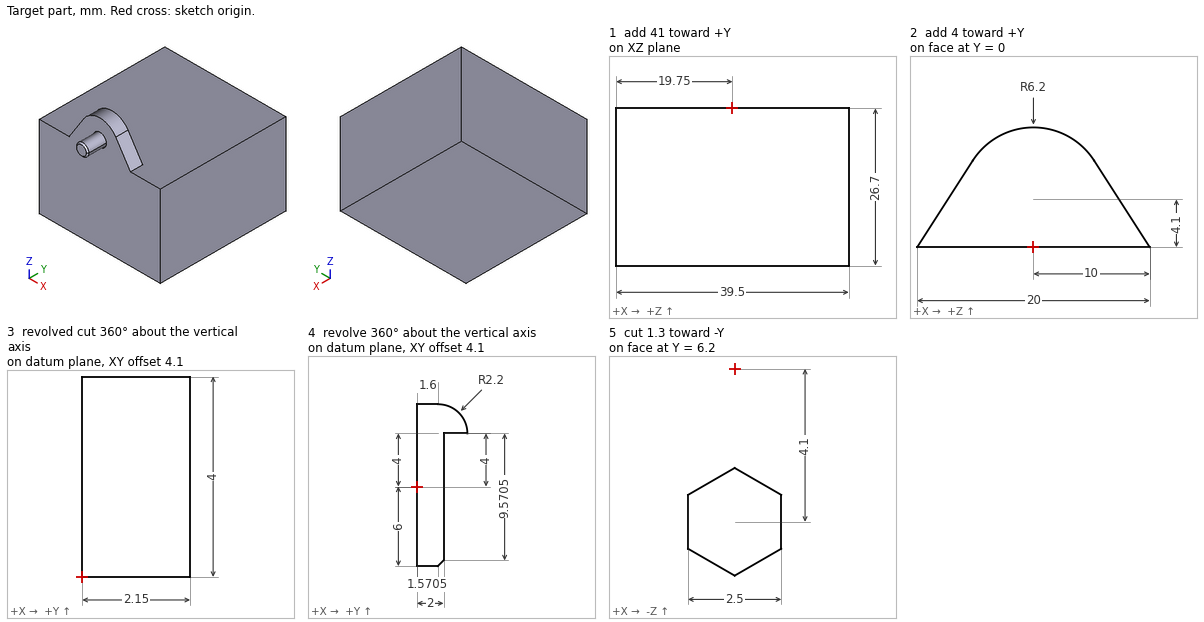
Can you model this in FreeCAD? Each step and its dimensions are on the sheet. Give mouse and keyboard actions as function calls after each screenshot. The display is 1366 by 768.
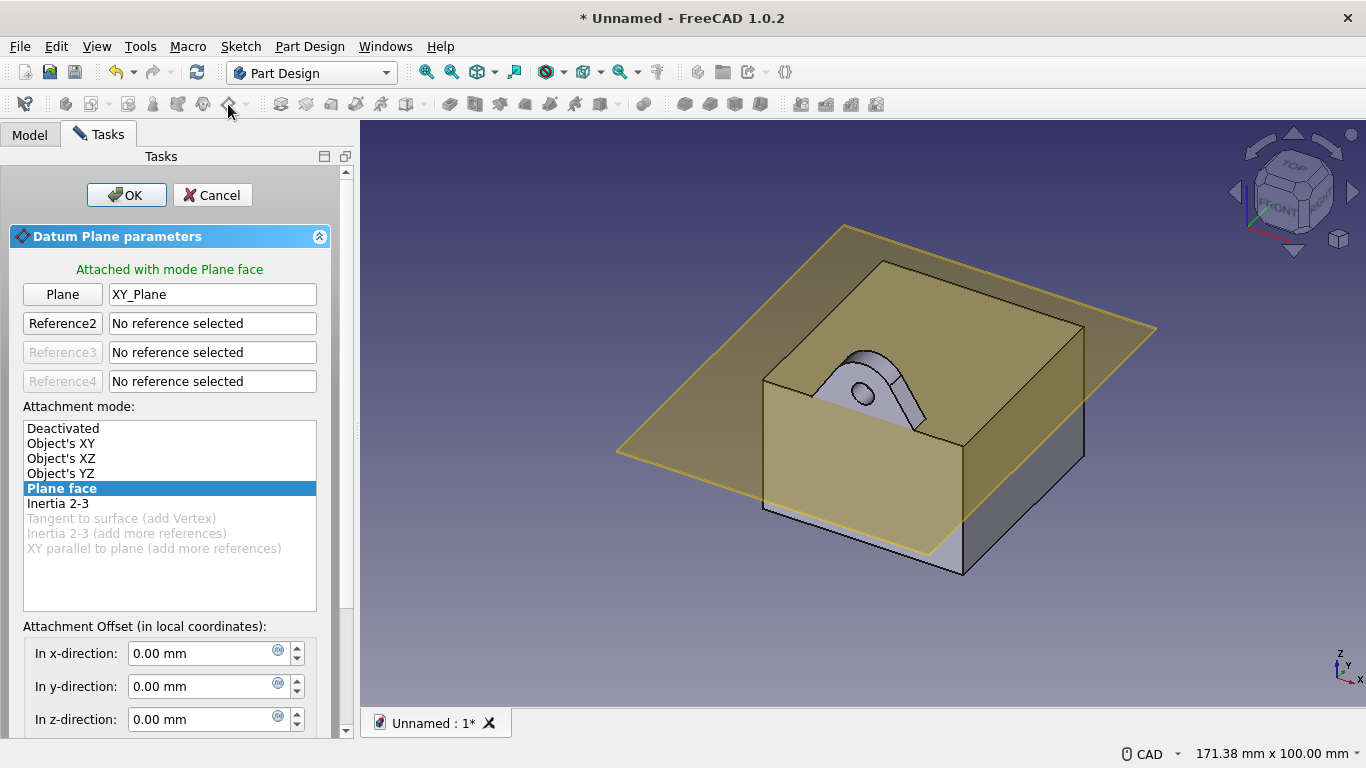
triple_click(210, 720)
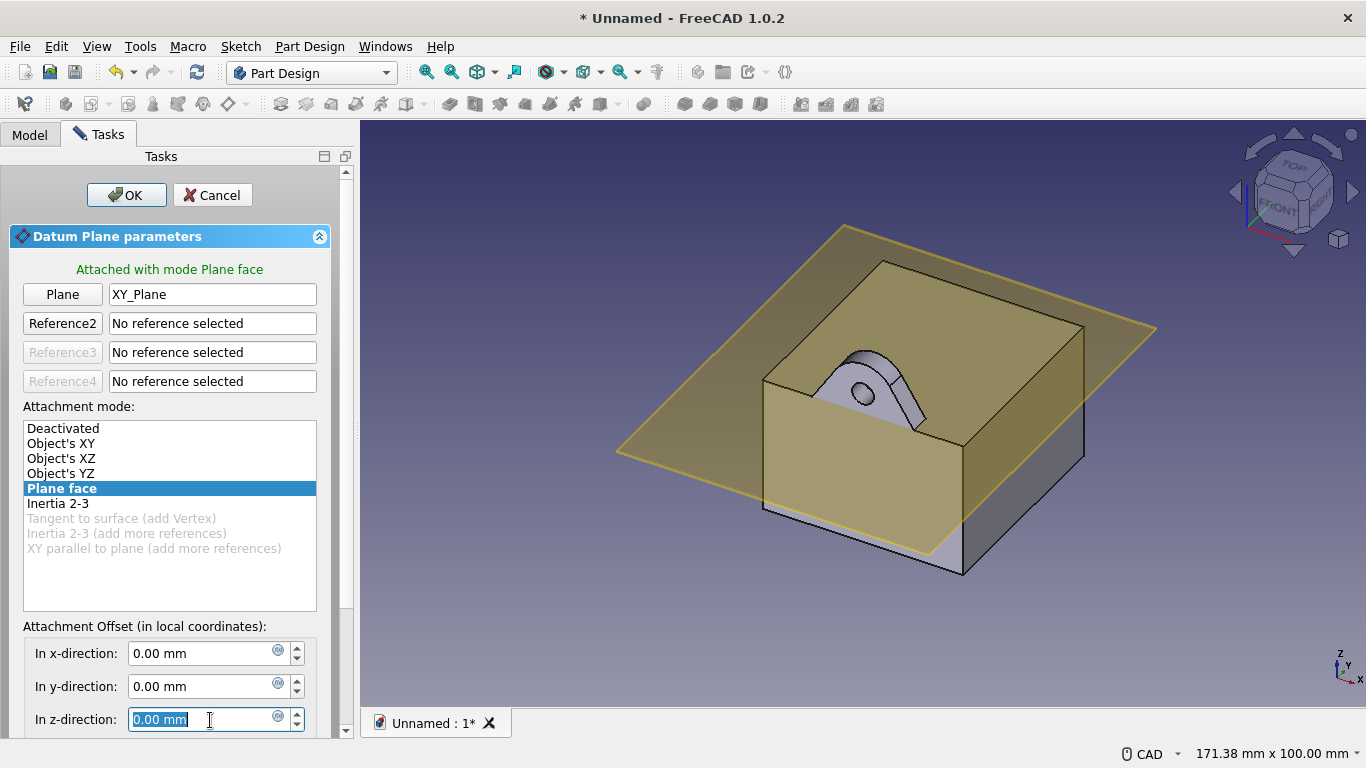
text(4.1)
key(Tab)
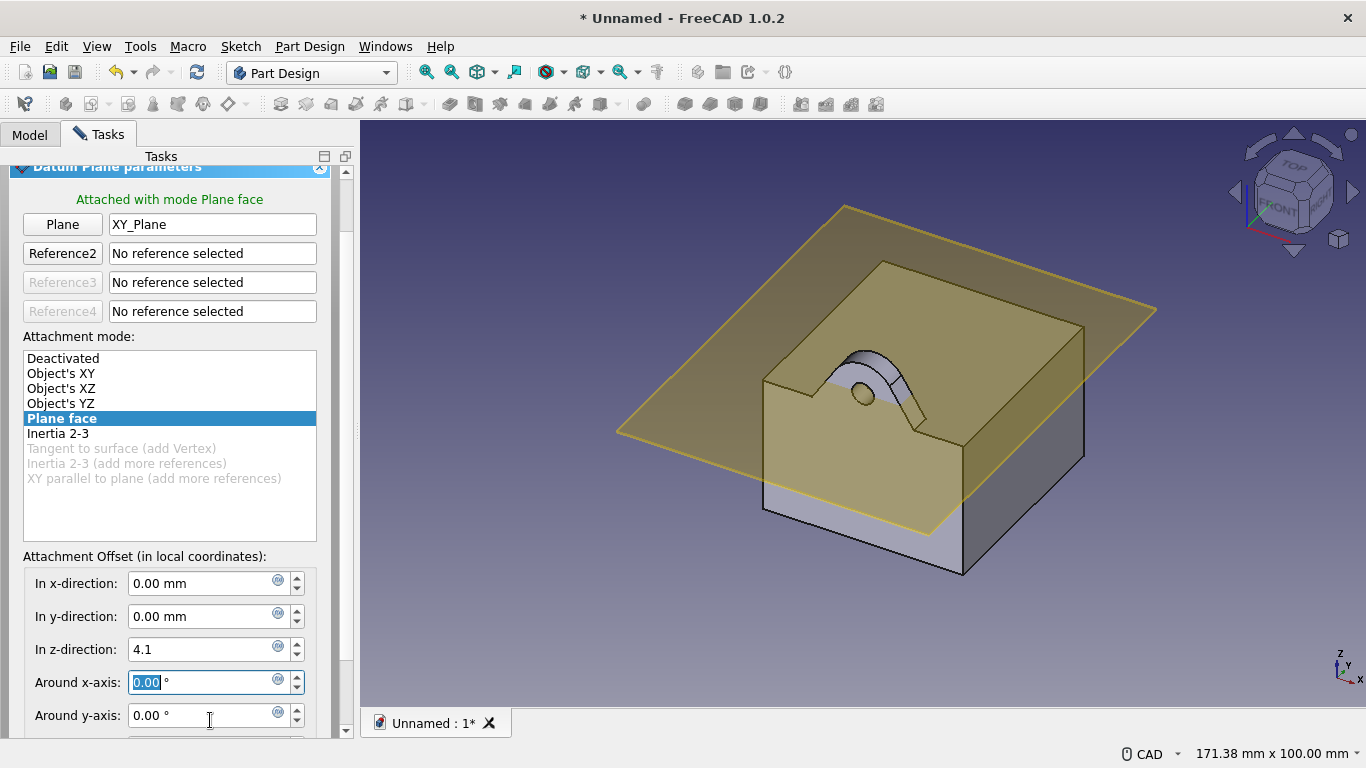
scroll(346, 452, up, 2)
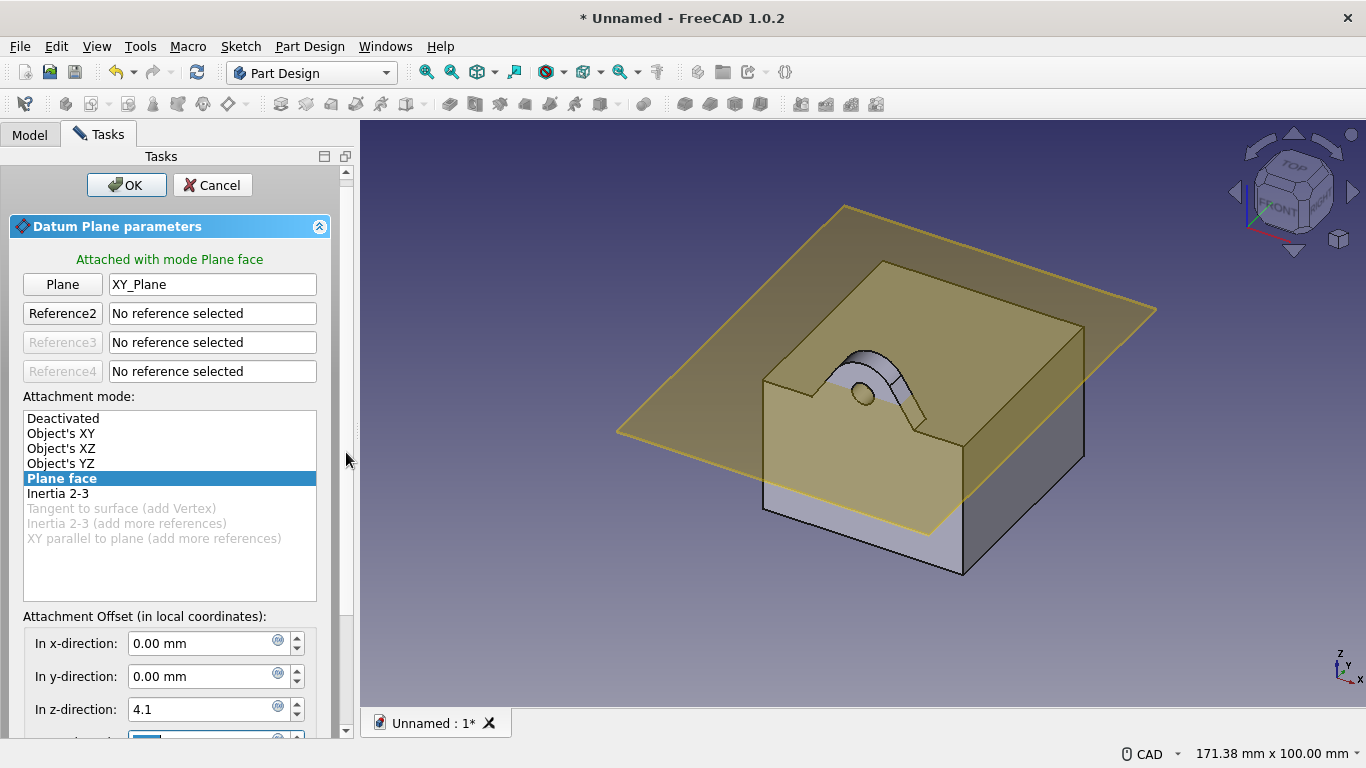
click(127, 195)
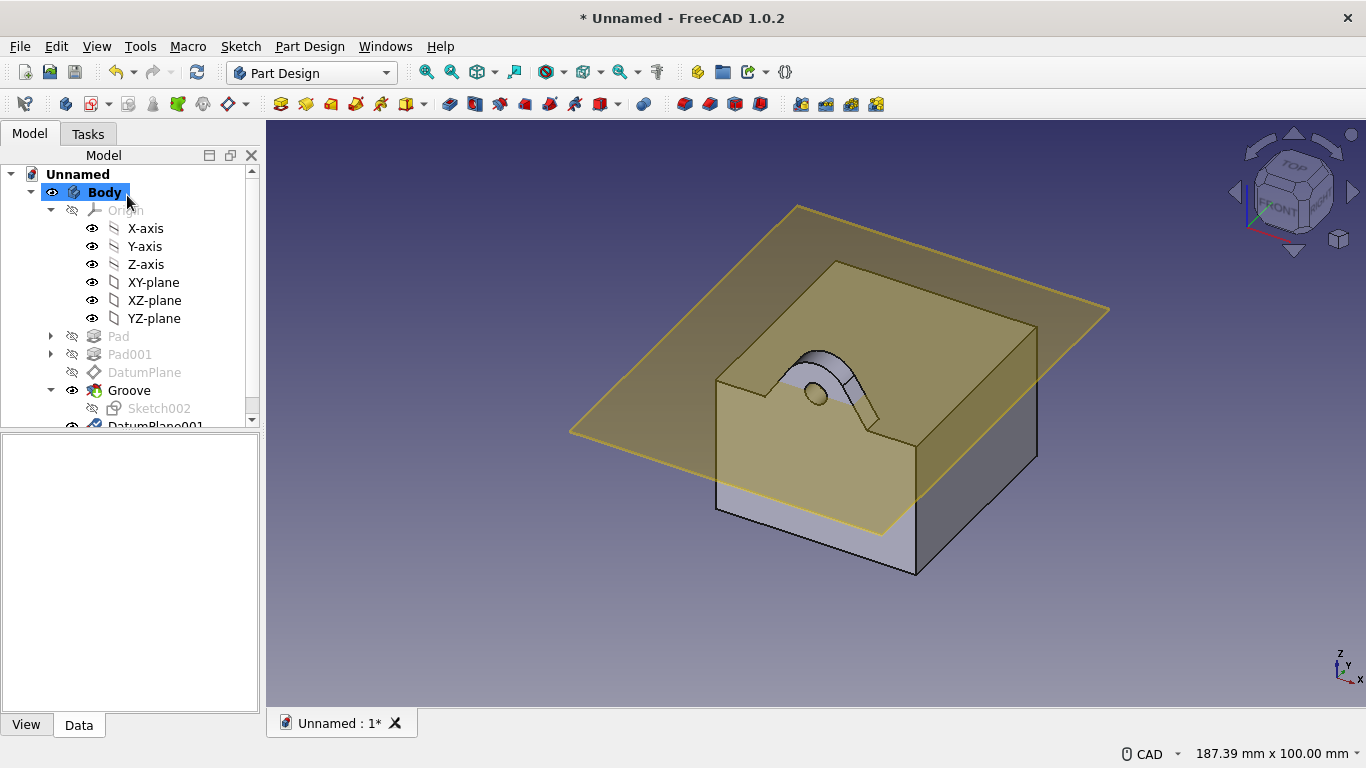
click(117, 426)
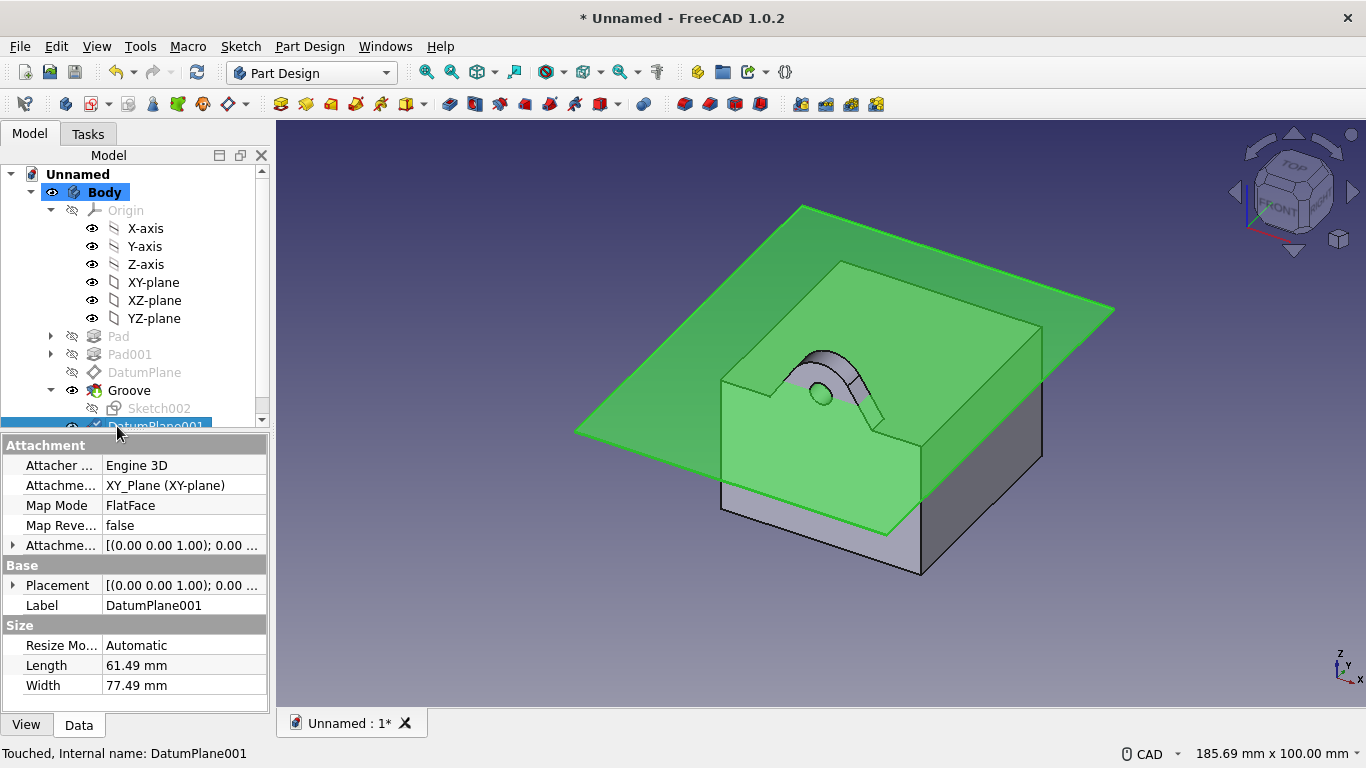
click(90, 104)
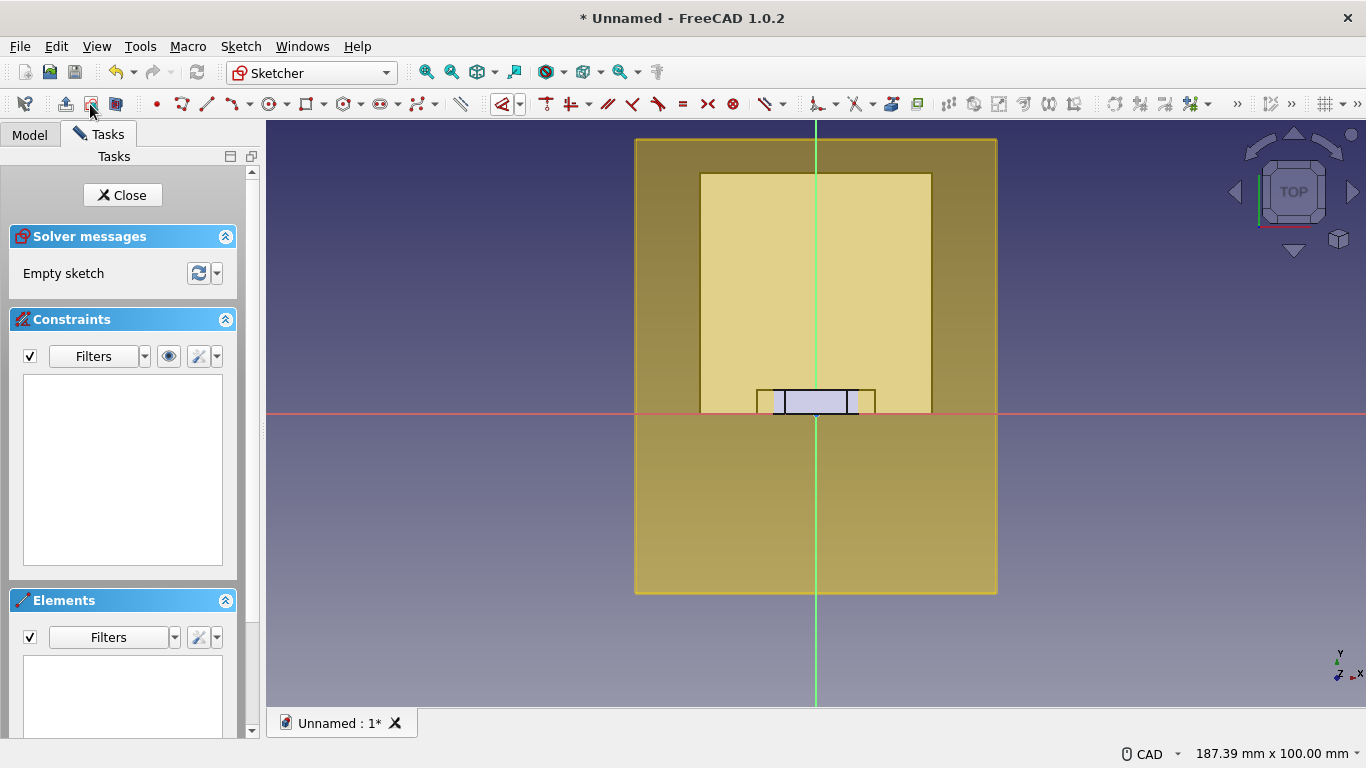
click(116, 104)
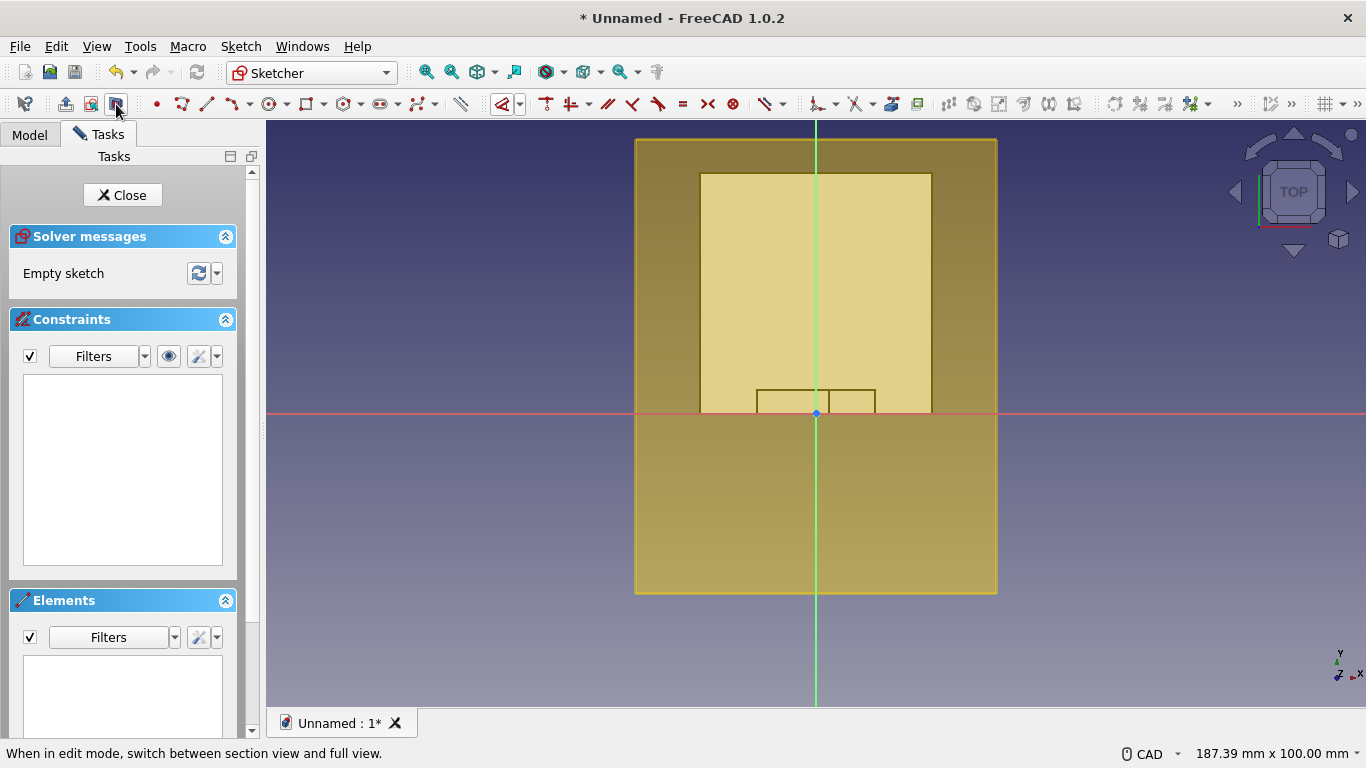
scroll(847, 413, up, 8)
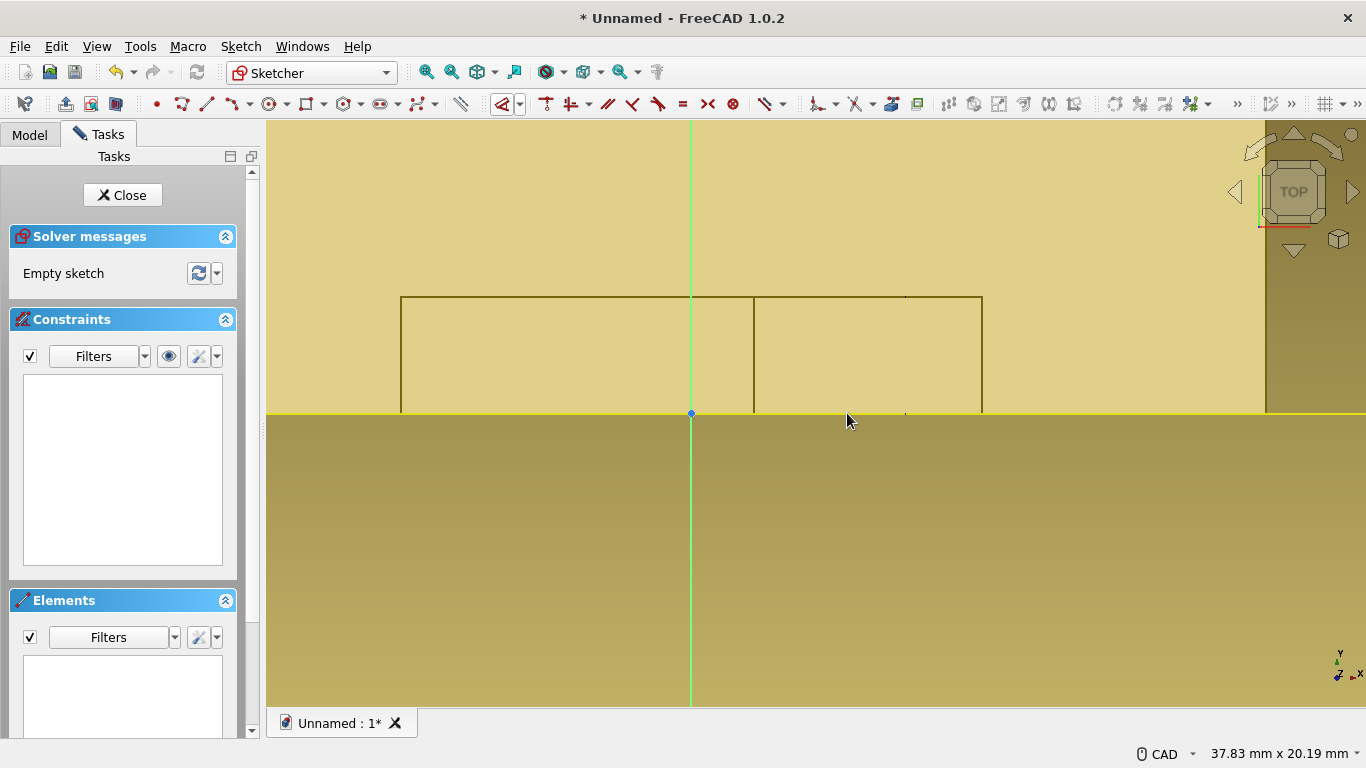
click(182, 104)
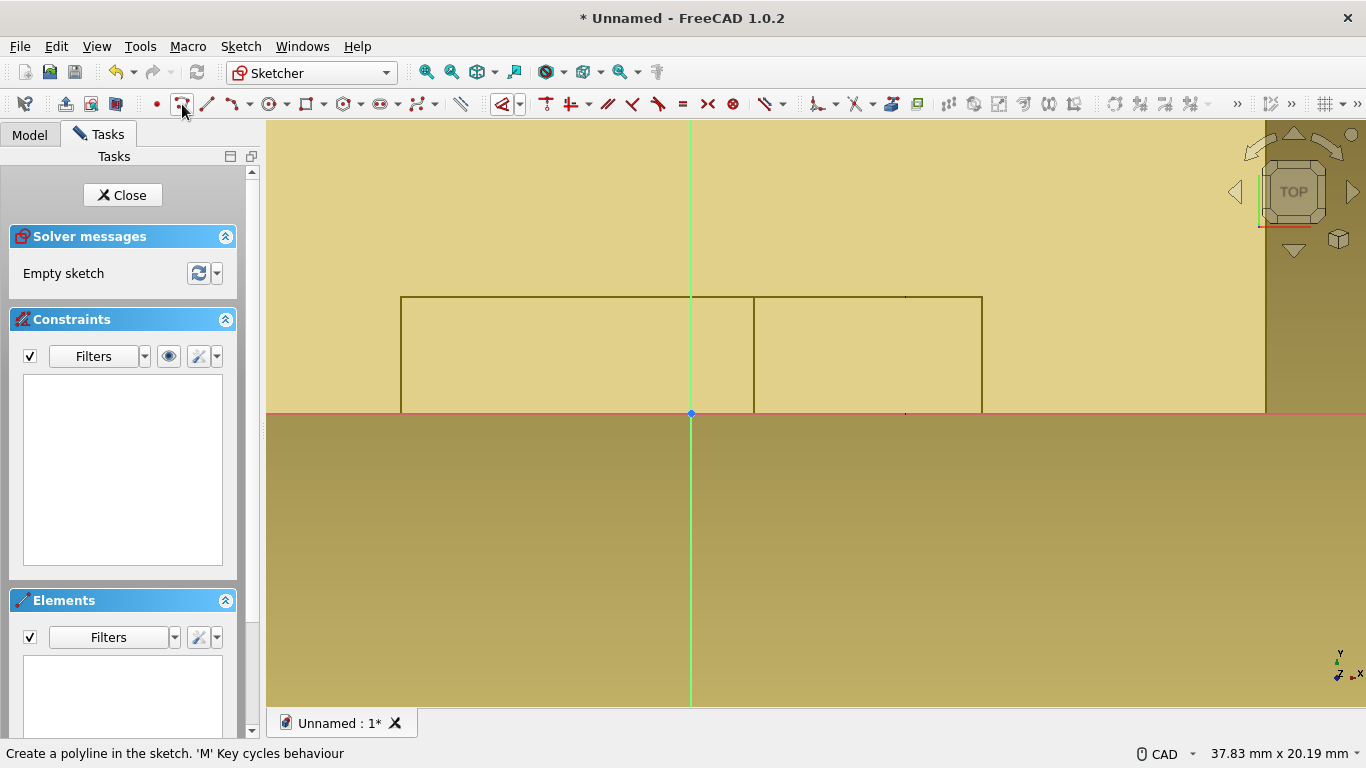
click(738, 233)
click(691, 233)
click(700, 588)
click(737, 588)
click(750, 575)
click(750, 297)
click(802, 297)
right_click(802, 297)